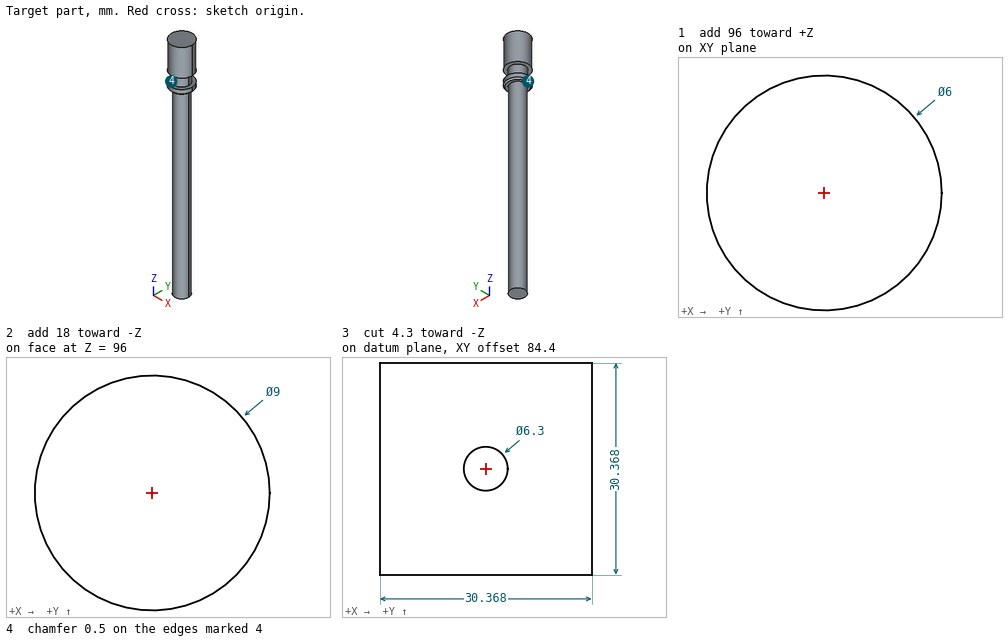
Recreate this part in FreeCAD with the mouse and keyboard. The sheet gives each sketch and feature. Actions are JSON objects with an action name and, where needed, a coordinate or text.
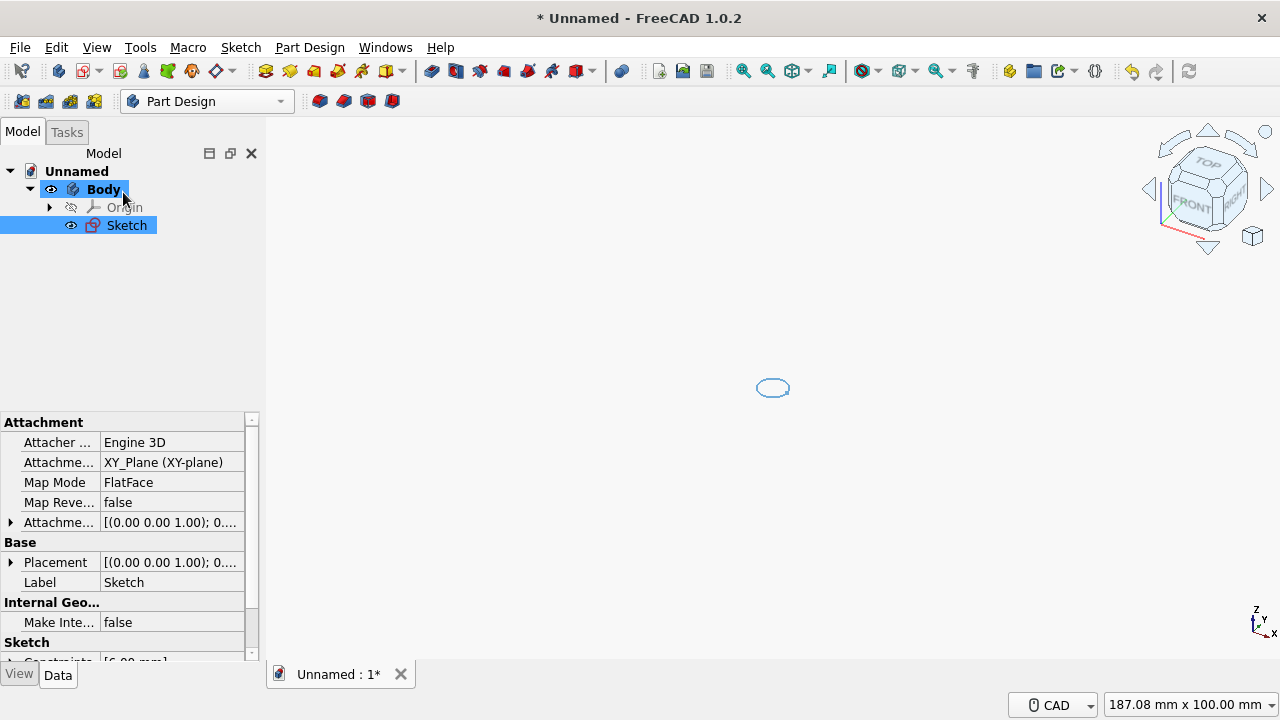
{"action": "left_click", "coordinate": [266, 72]}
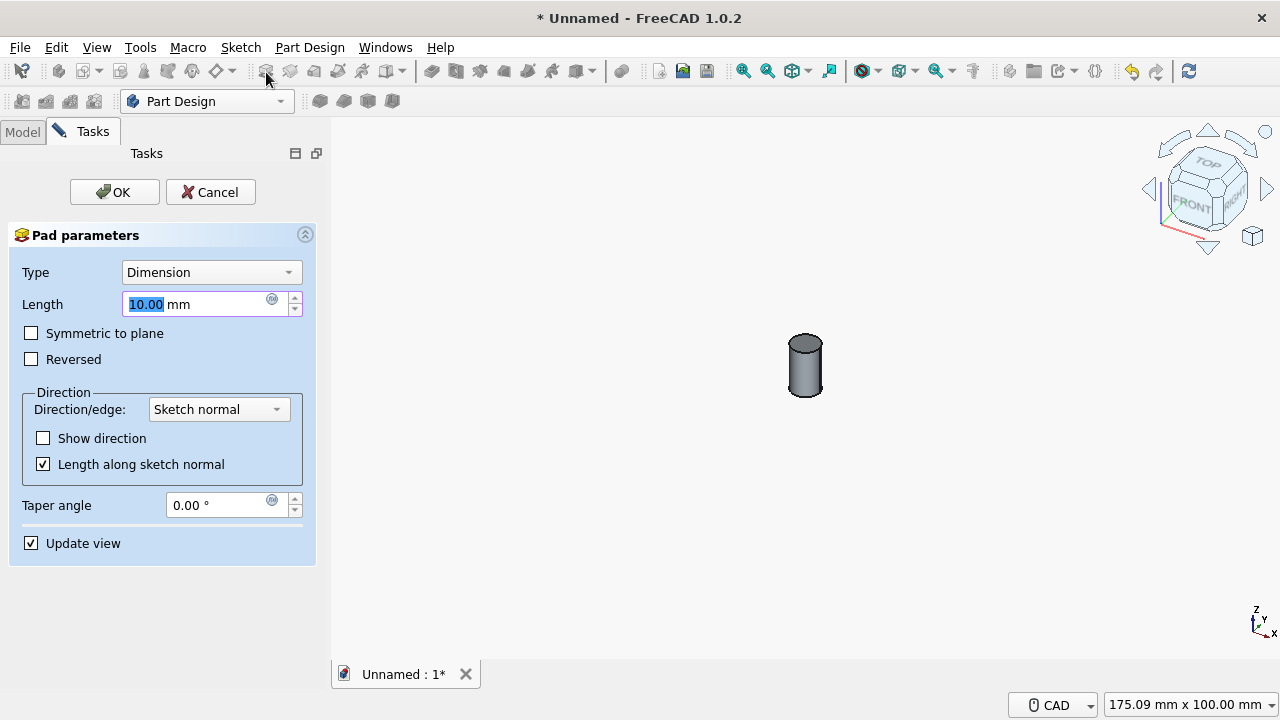
{"action": "type", "text": "96"}
{"action": "key", "text": "Tab"}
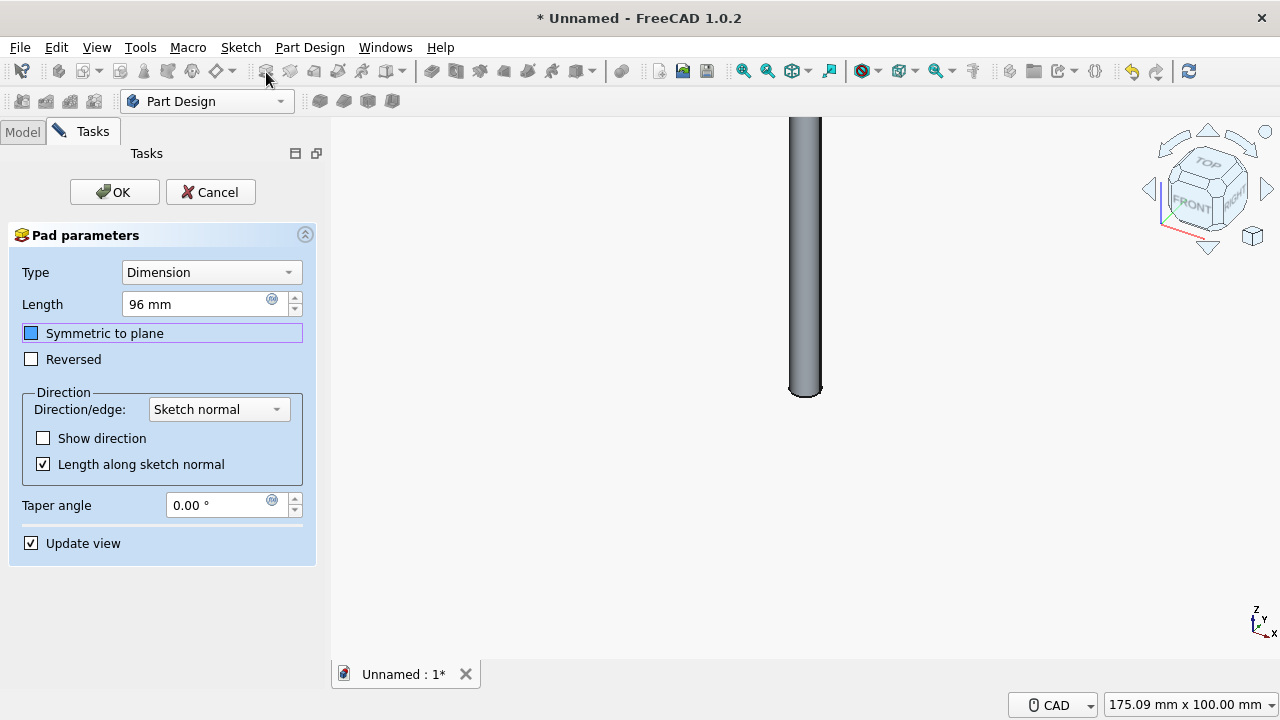
{"action": "left_click", "coordinate": [115, 192]}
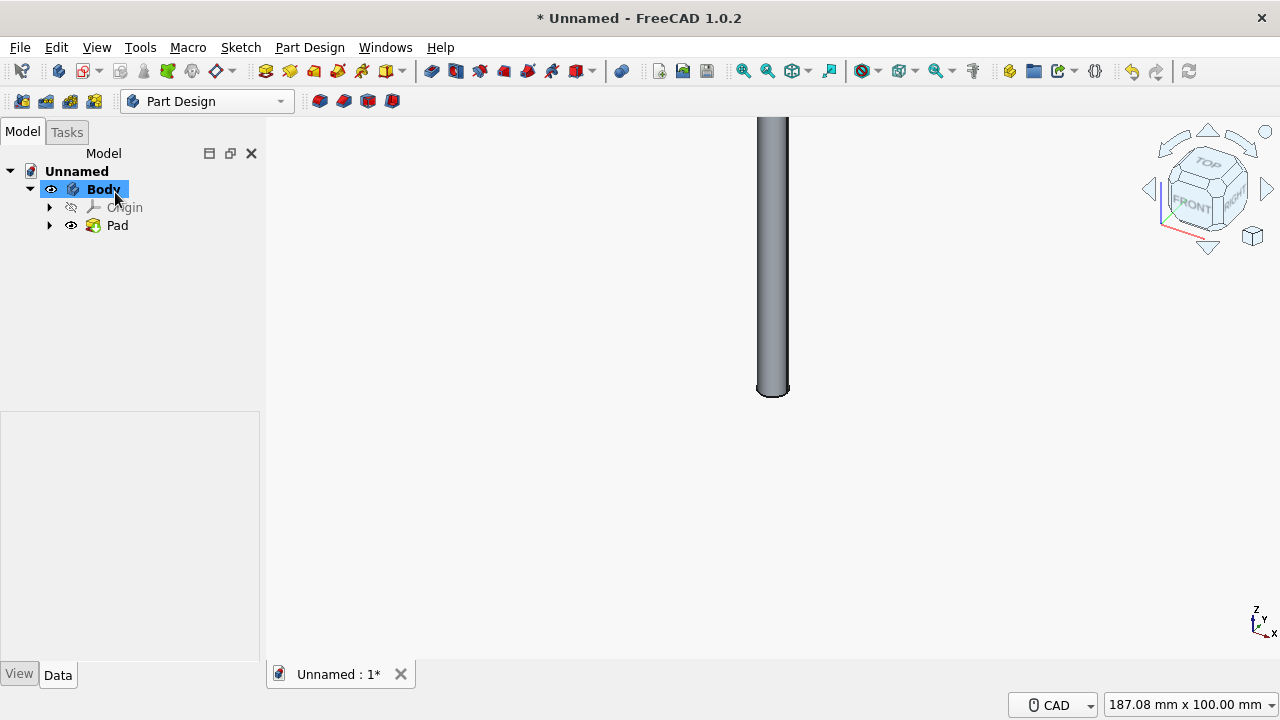
{"action": "key", "text": "v f"}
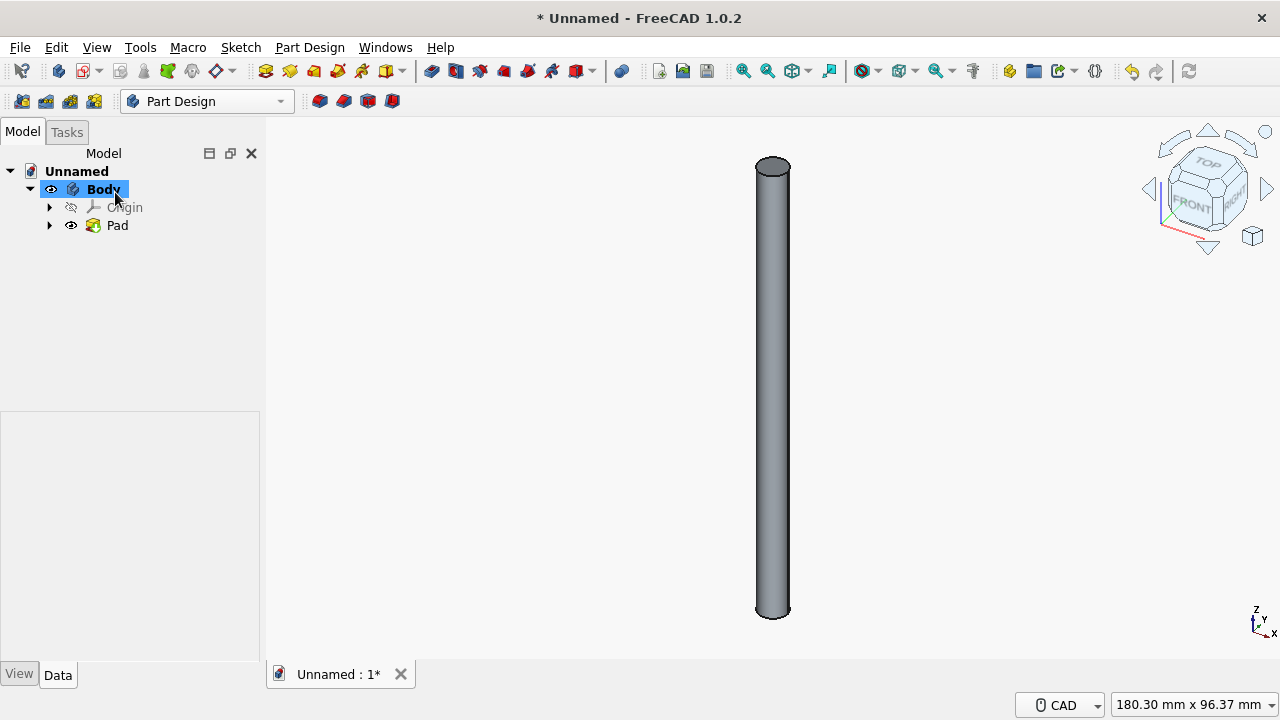
{"action": "left_click", "coordinate": [773, 166]}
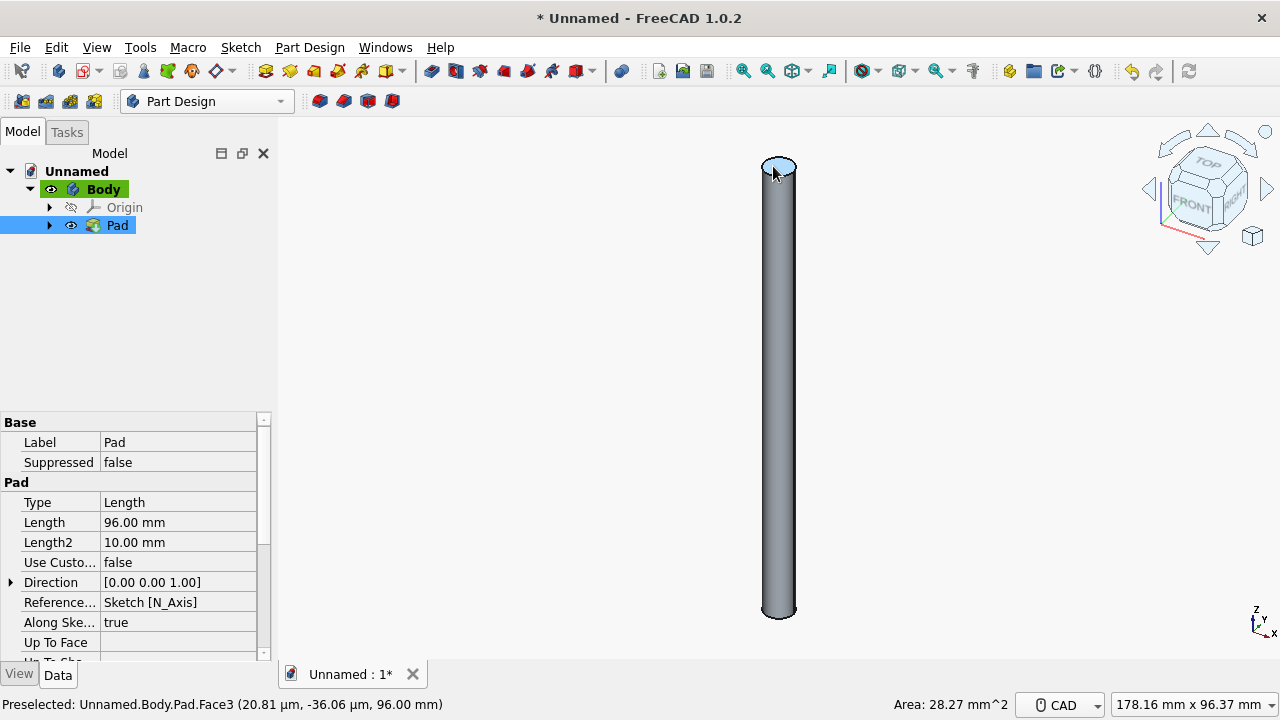
{"action": "left_click", "coordinate": [84, 72]}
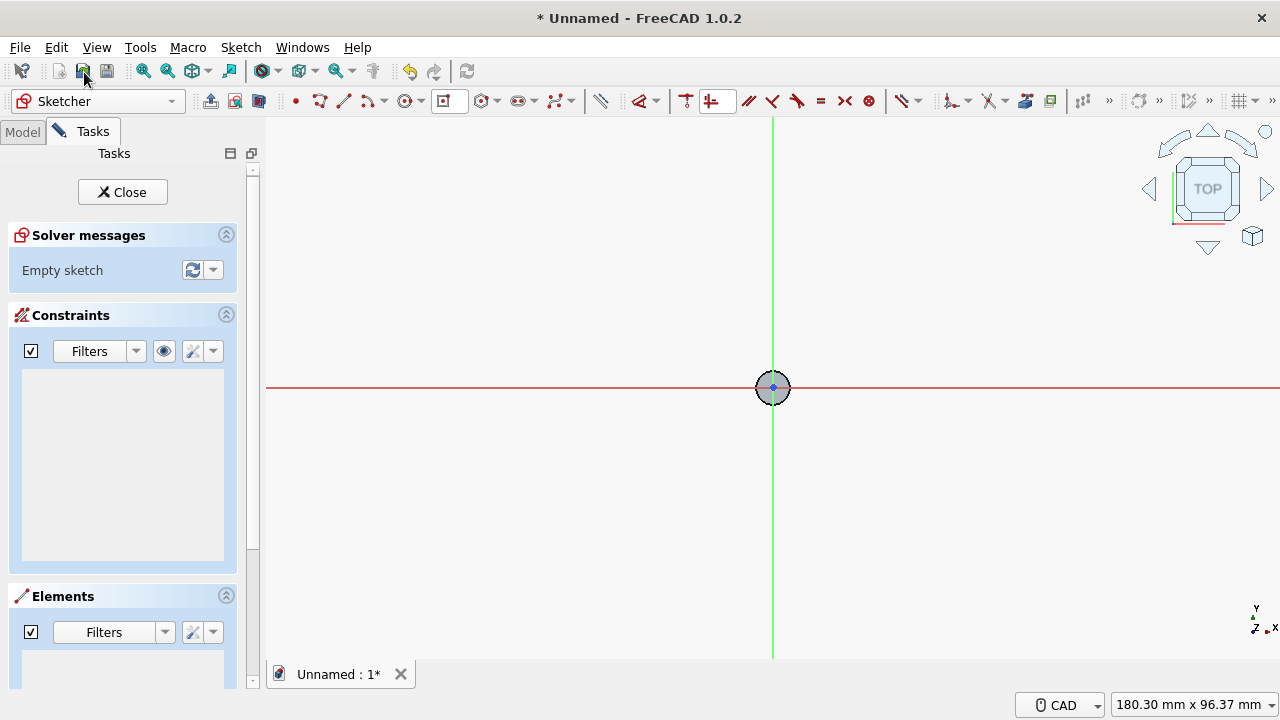
{"action": "scroll", "coordinate": [784, 388], "scroll_direction": "up", "scroll_amount": 10}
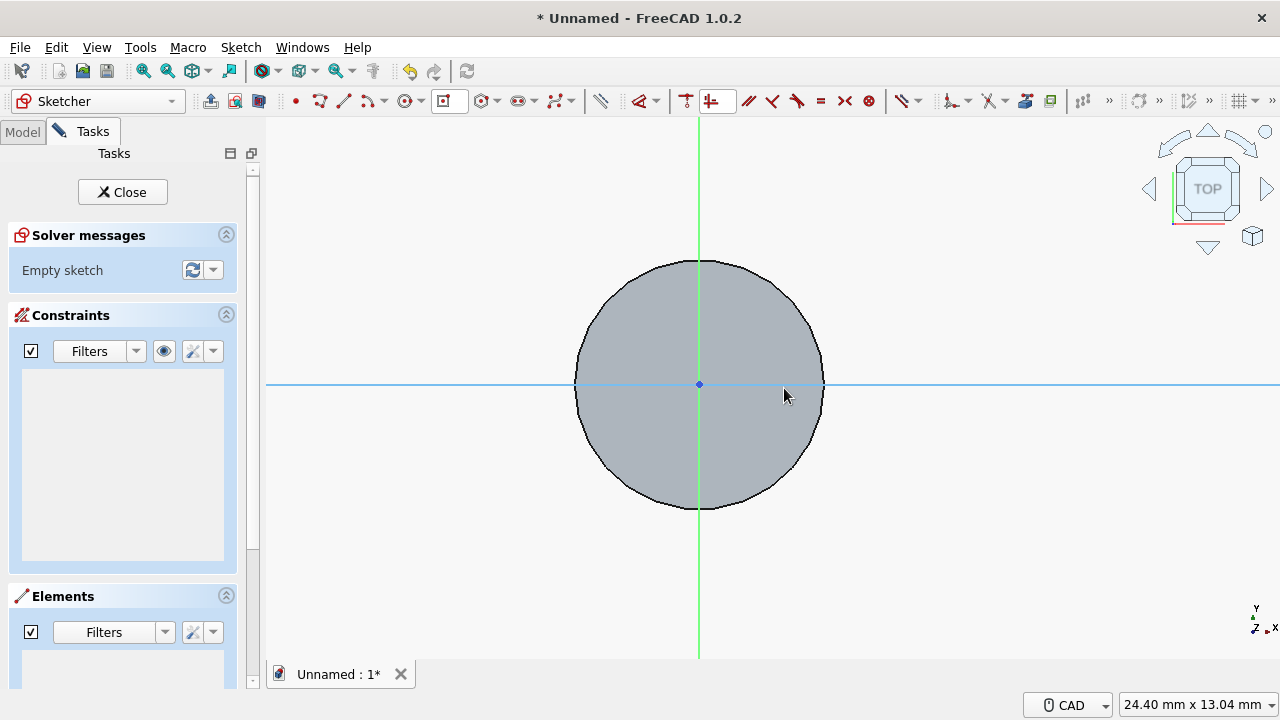
{"action": "key", "text": "g c"}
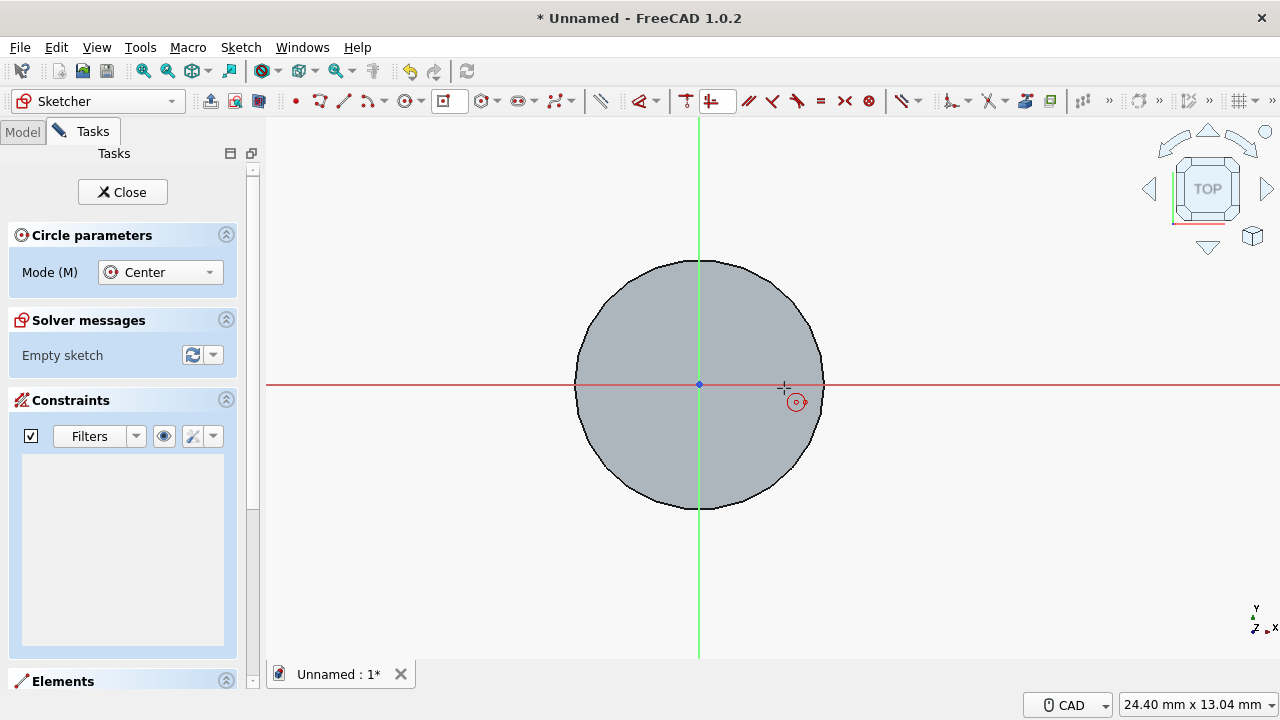
{"action": "left_click", "coordinate": [699, 385]}
{"action": "left_click", "coordinate": [832, 253]}
{"action": "key", "text": "Escape"}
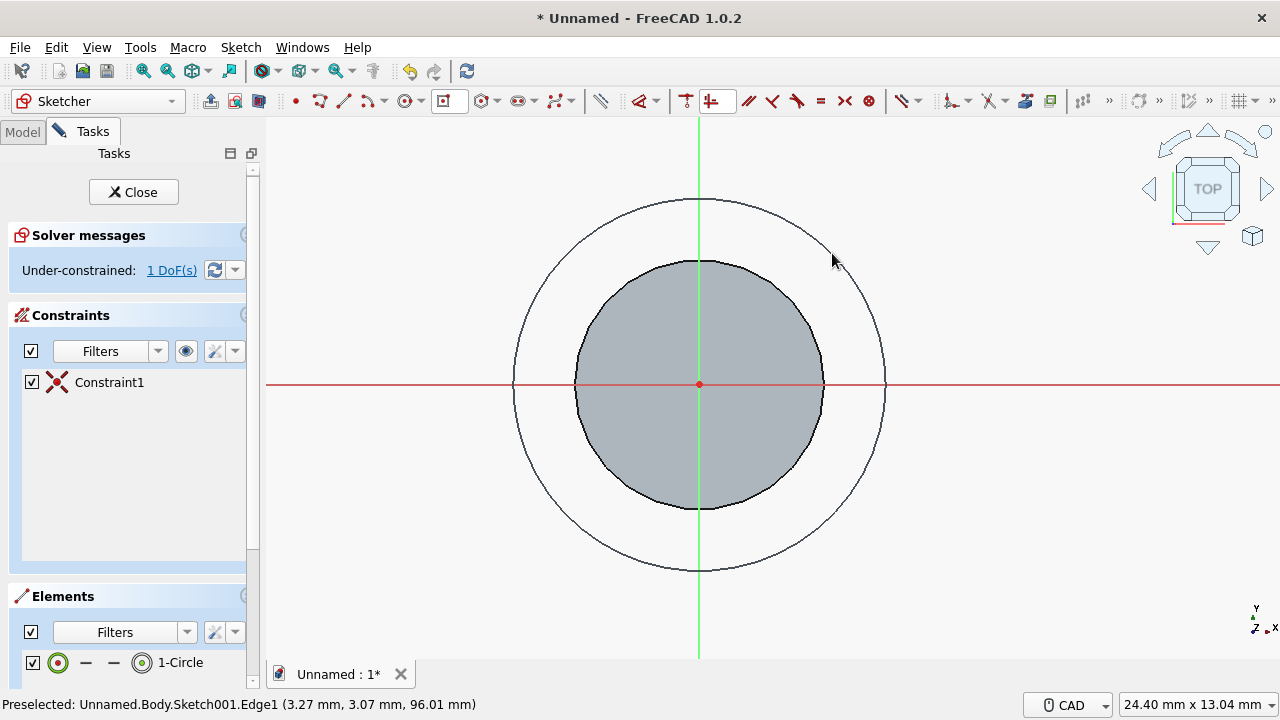
{"action": "left_click", "coordinate": [640, 102]}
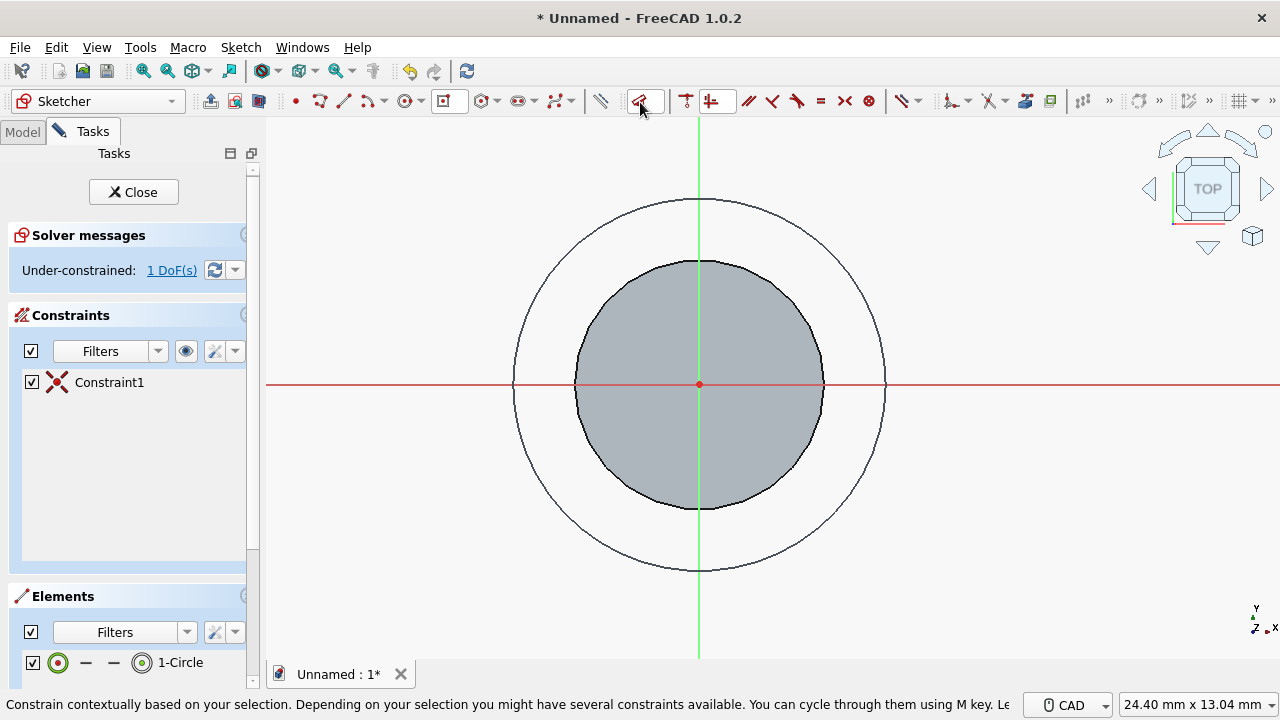
{"action": "left_click", "coordinate": [831, 253]}
{"action": "left_click", "coordinate": [854, 230]}